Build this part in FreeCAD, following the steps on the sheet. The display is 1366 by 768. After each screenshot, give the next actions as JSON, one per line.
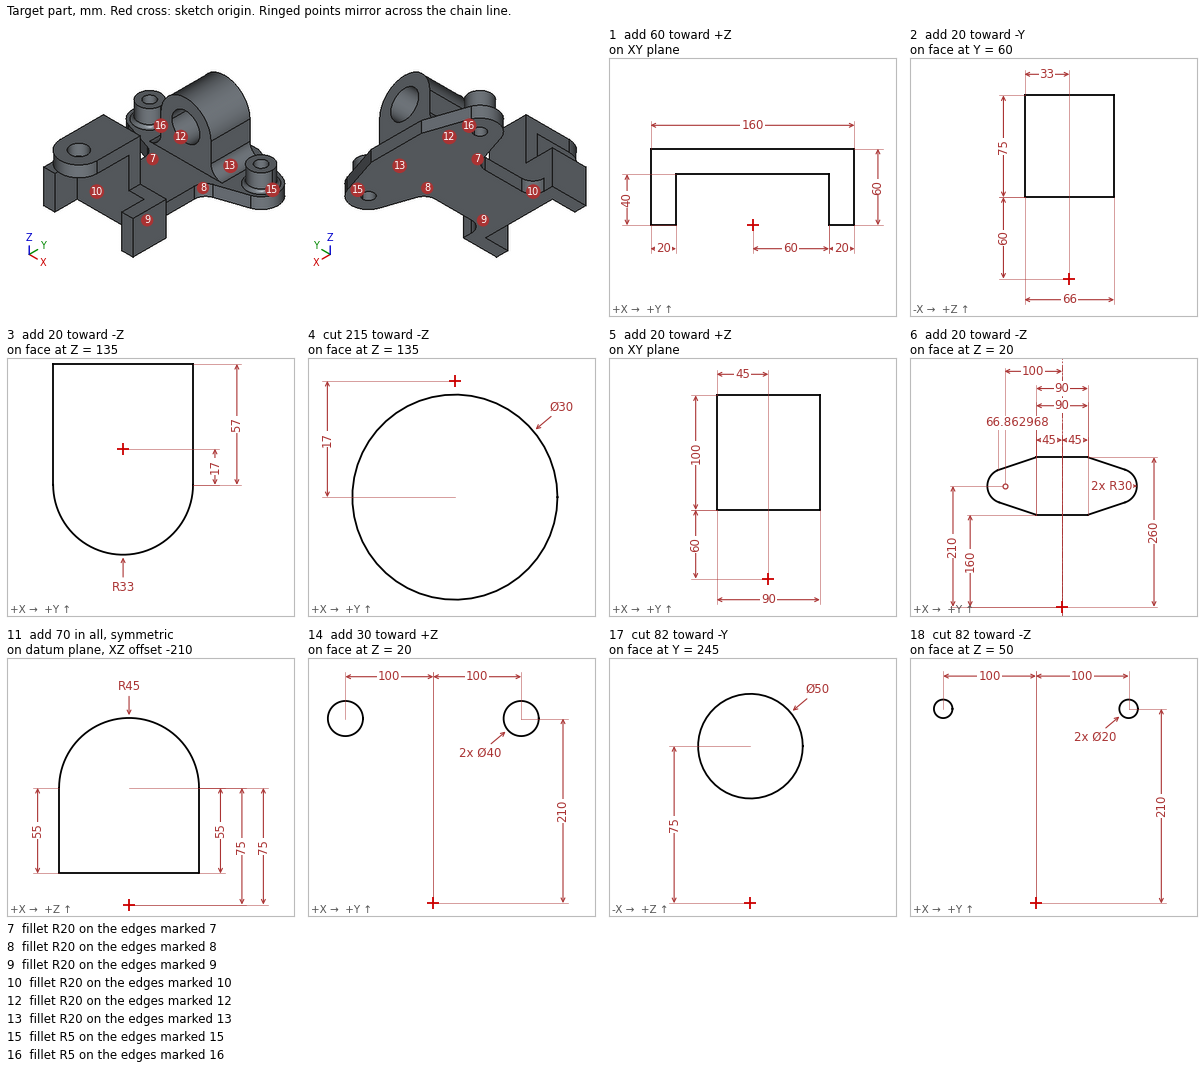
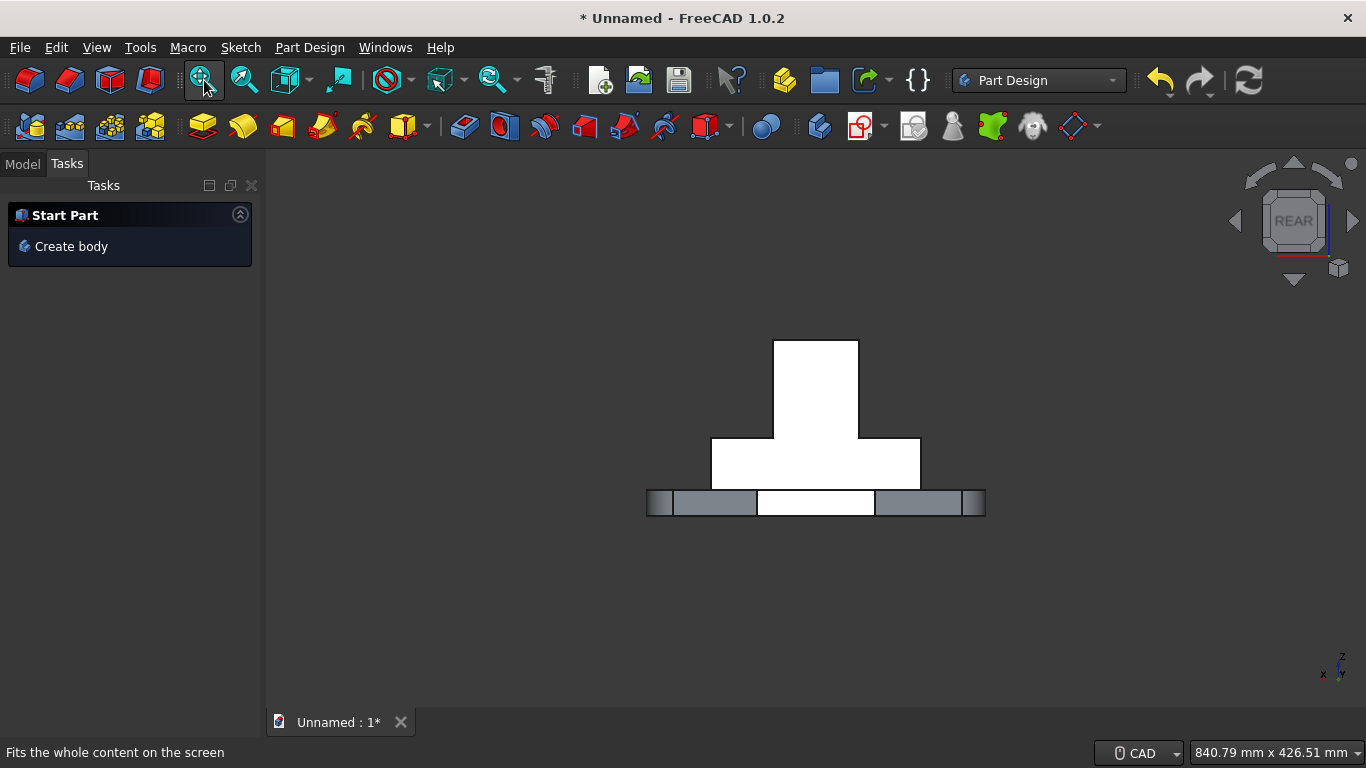
{"action": "key", "text": "6"}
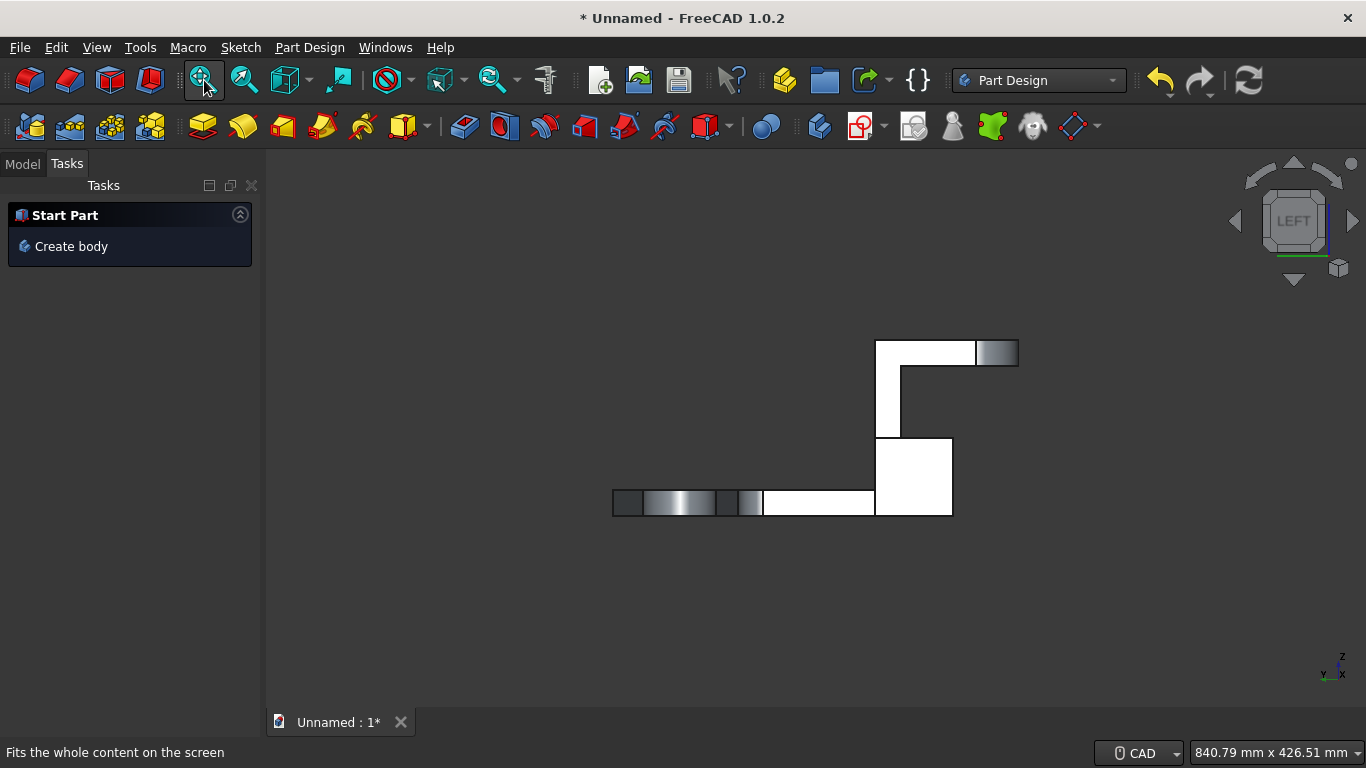
{"action": "left_click", "coordinate": [204, 80]}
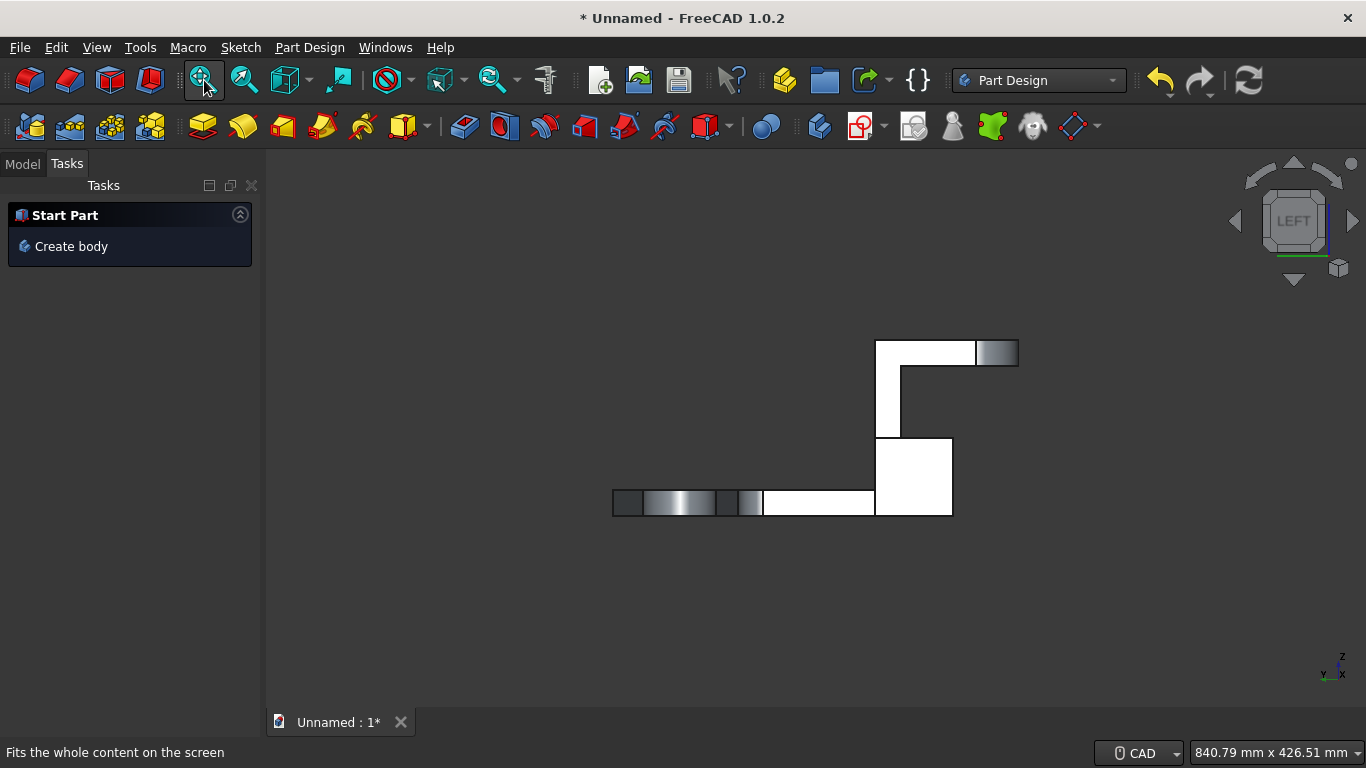
{"action": "key", "text": "v 3"}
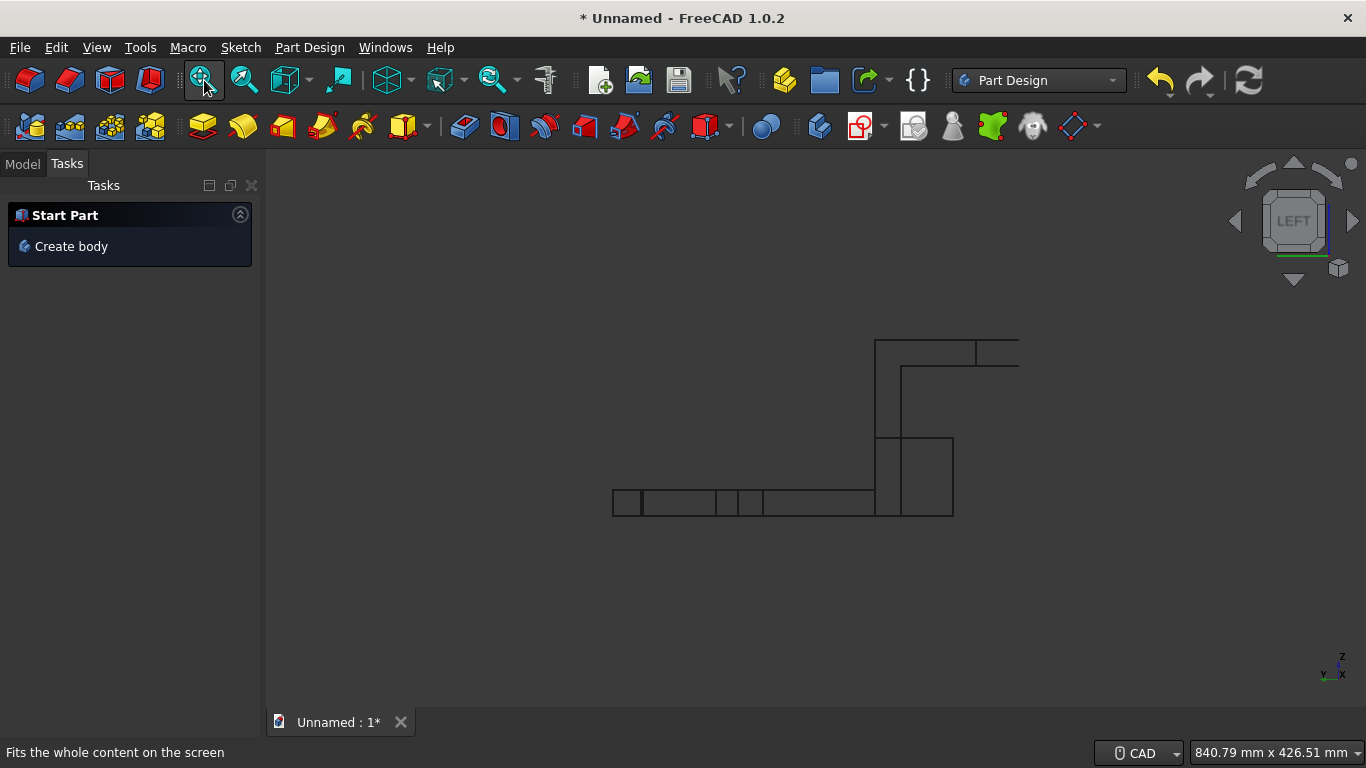
{"action": "key", "text": "0"}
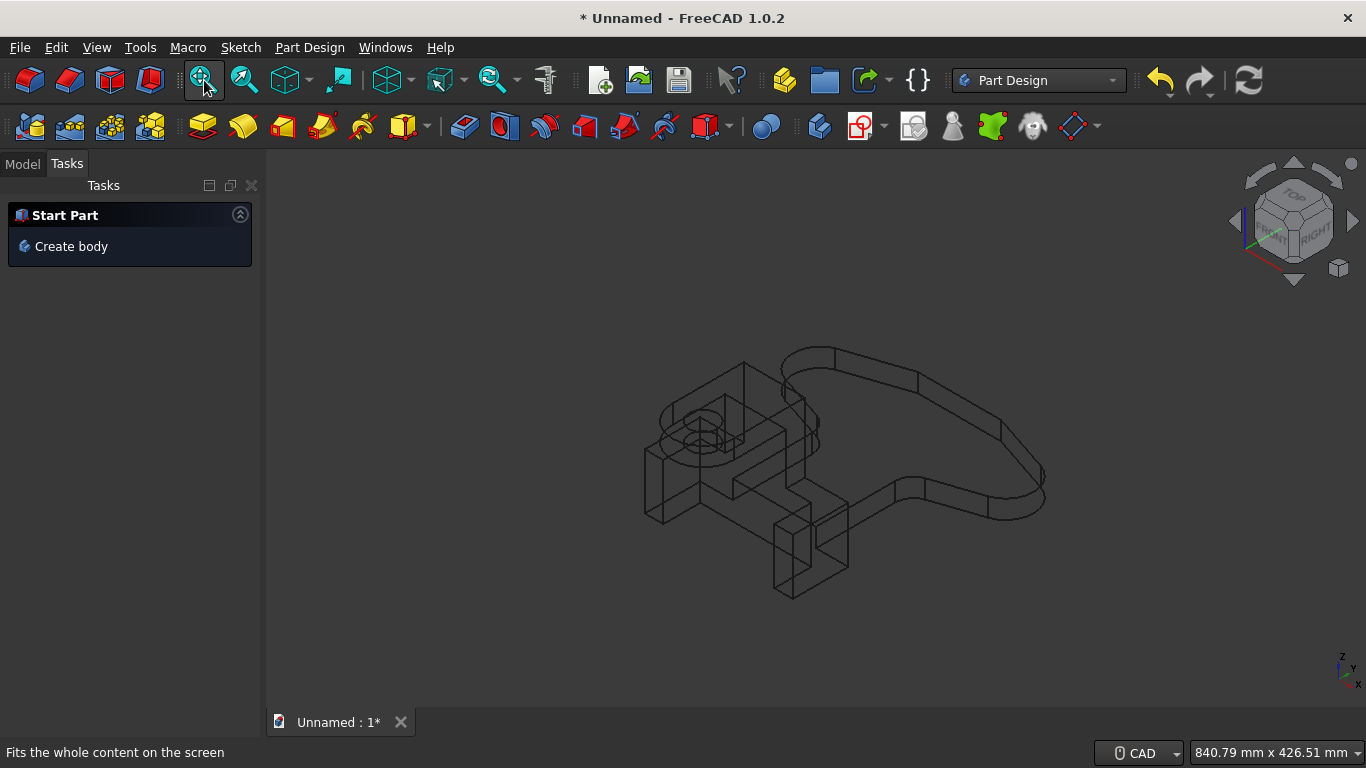
{"action": "scroll", "coordinate": [816, 536], "scroll_direction": "up", "scroll_amount": 6}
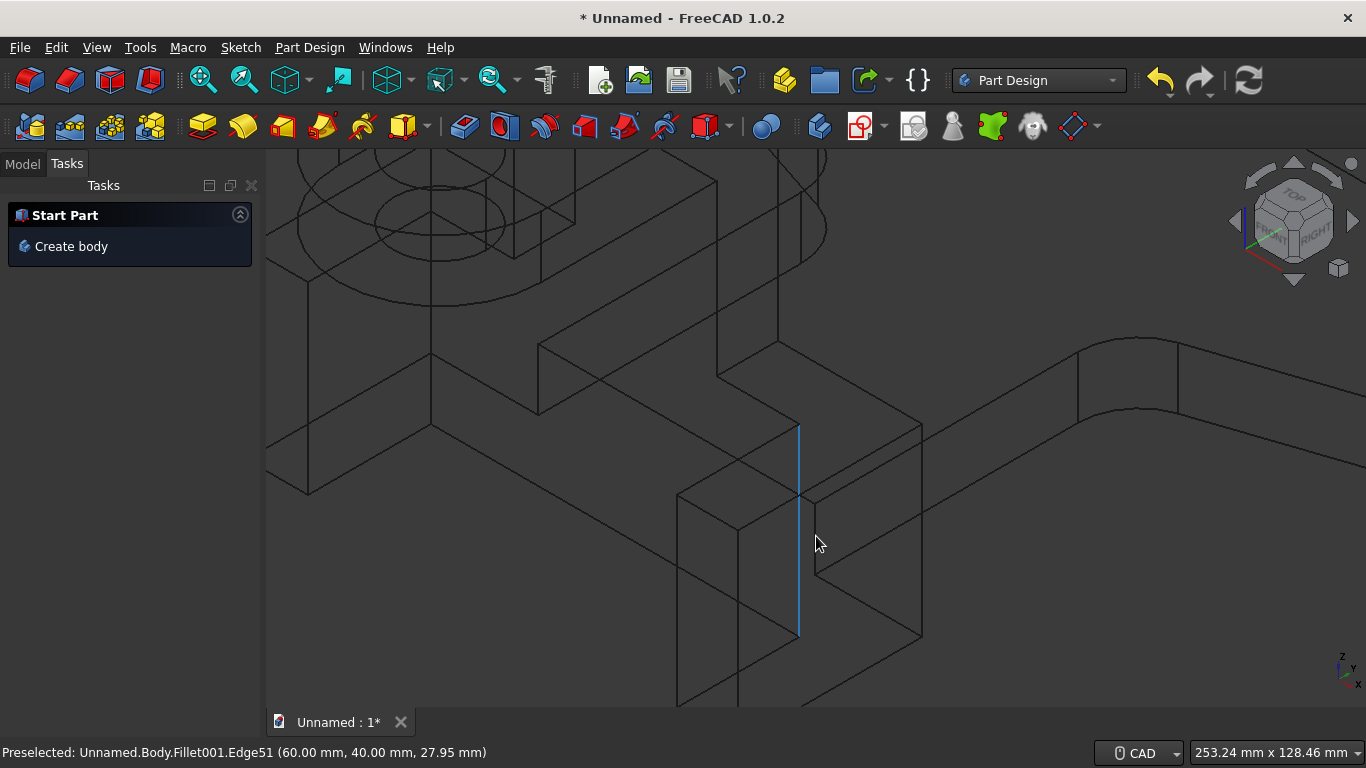
{"action": "left_click", "coordinate": [815, 538]}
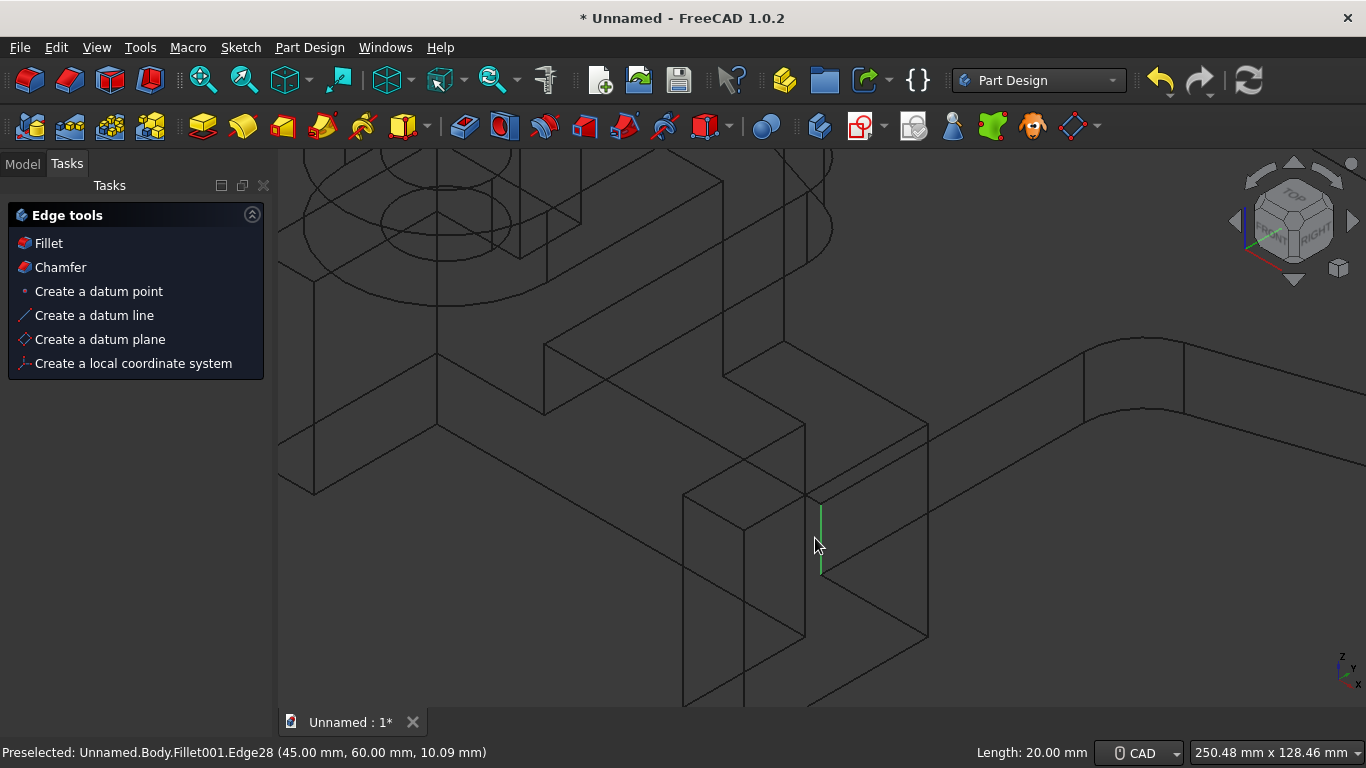
{"action": "key", "text": "v 1"}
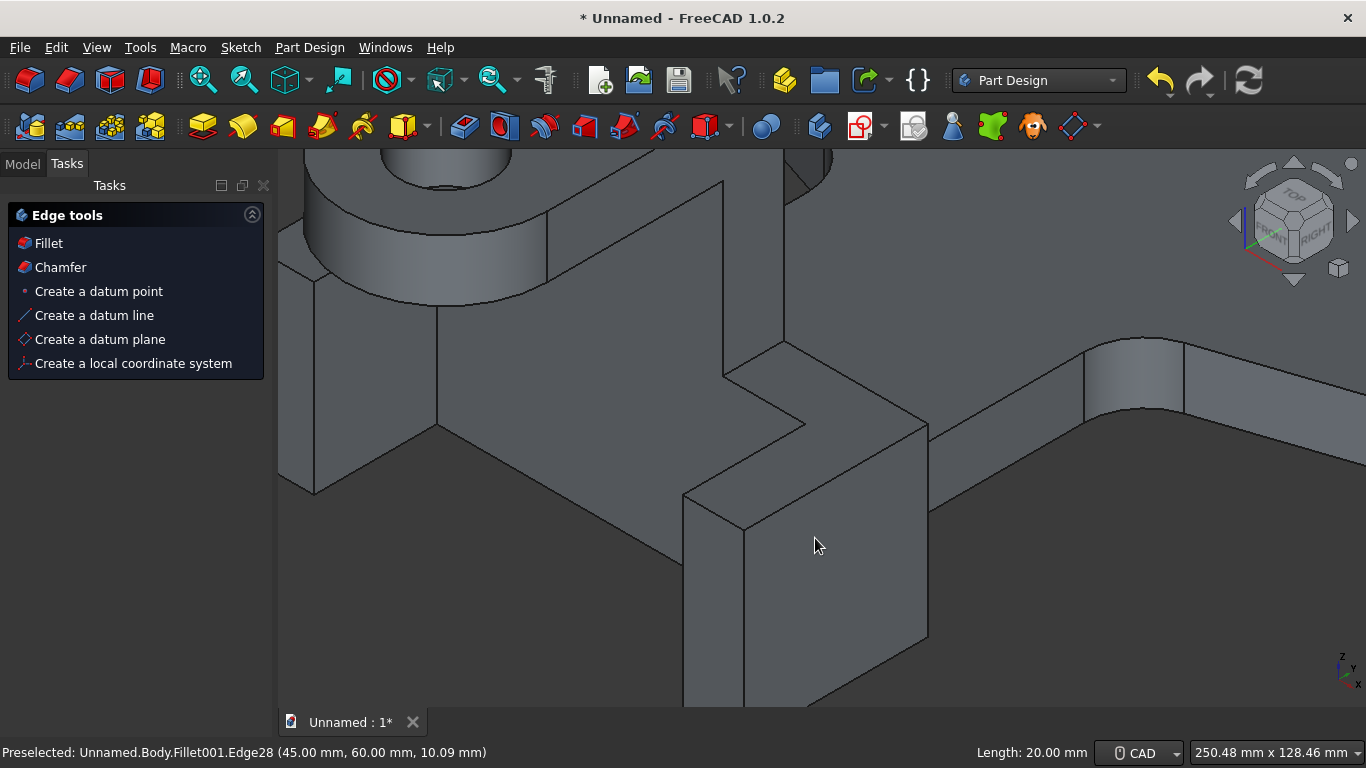
{"action": "left_click", "coordinate": [30, 80]}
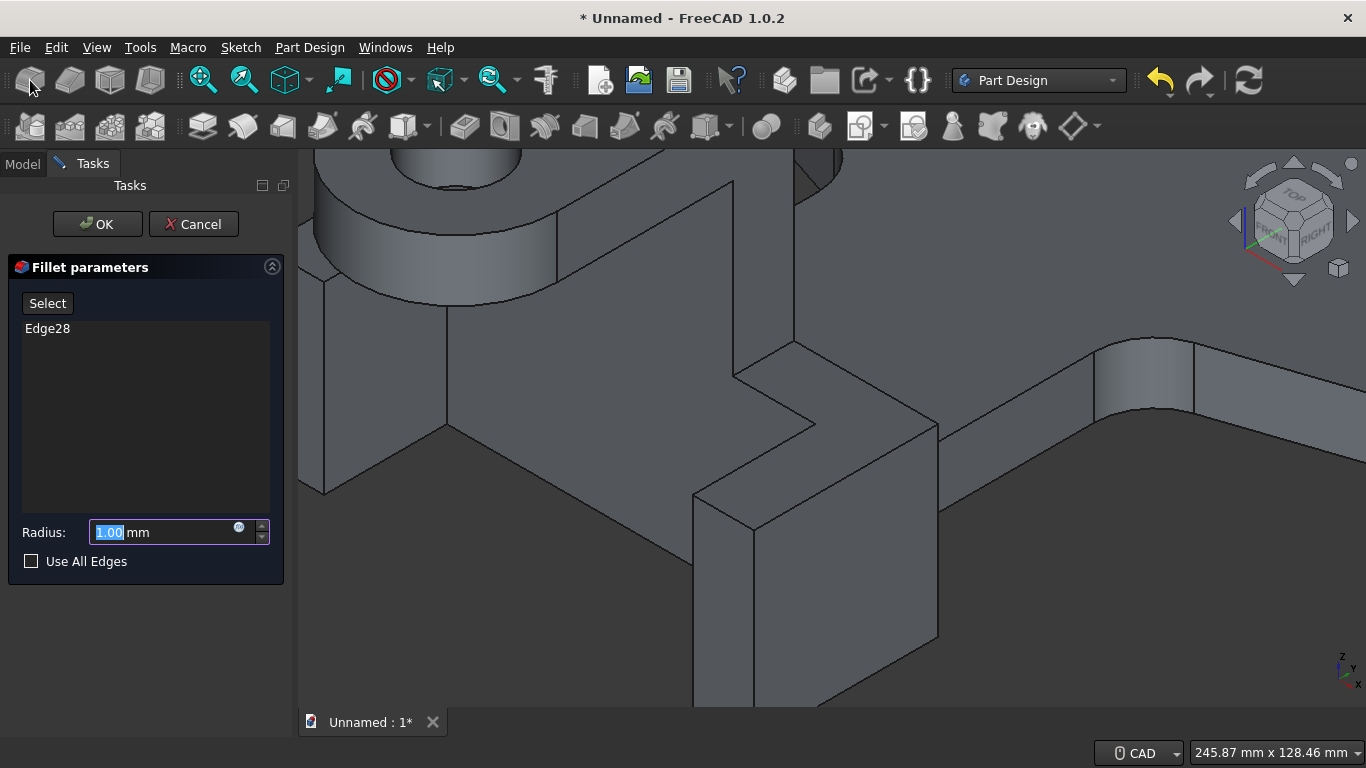
{"action": "type", "text": "20"}
{"action": "key", "text": "Tab"}